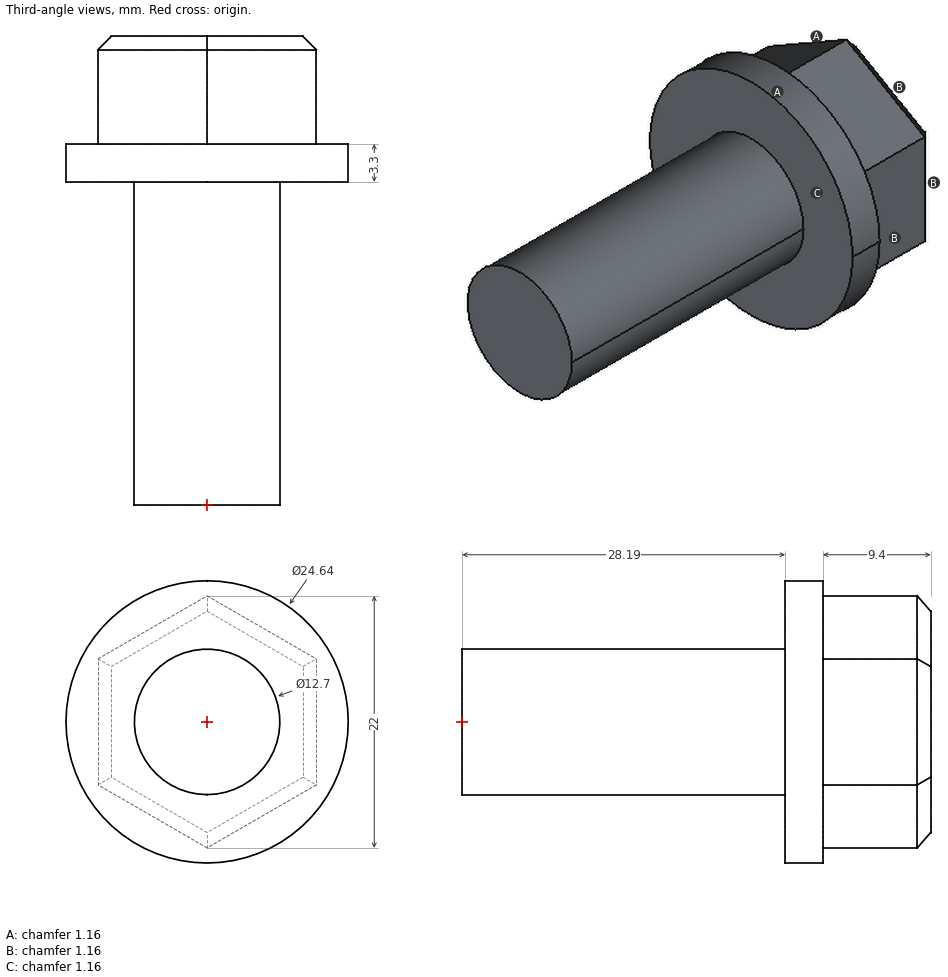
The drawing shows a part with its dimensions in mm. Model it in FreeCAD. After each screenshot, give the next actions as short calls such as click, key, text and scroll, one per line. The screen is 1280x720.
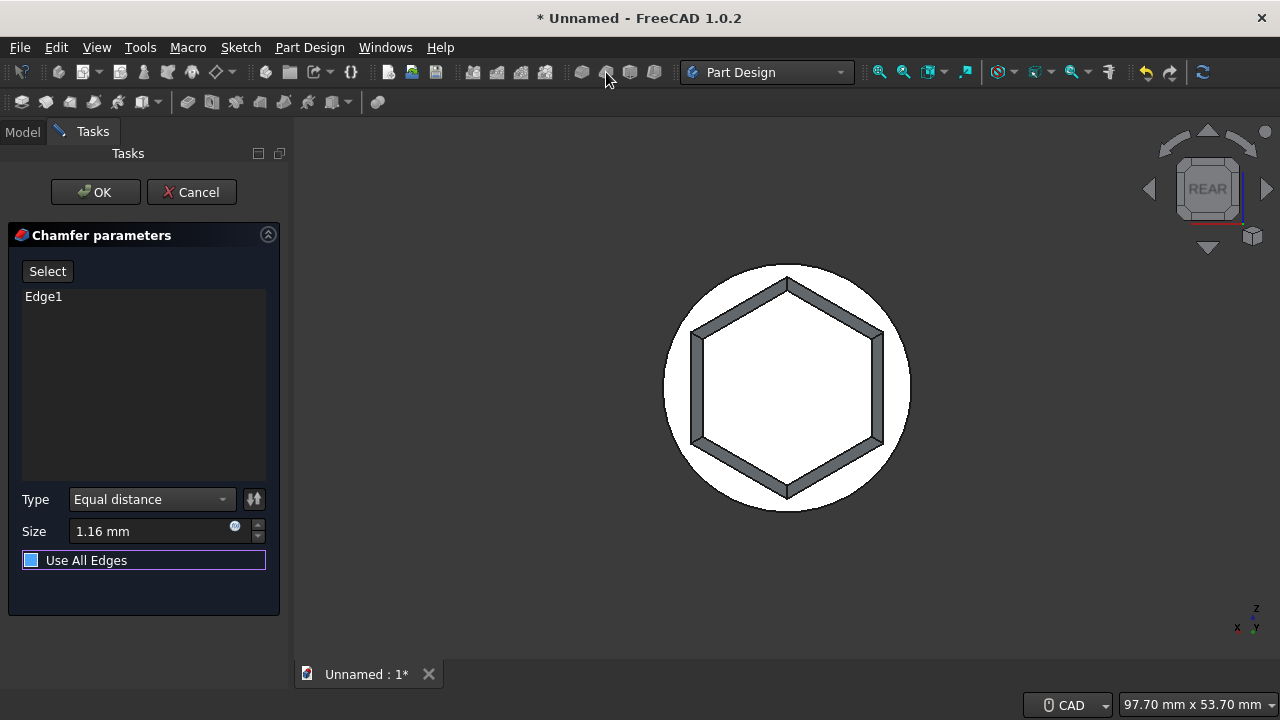
click(96, 192)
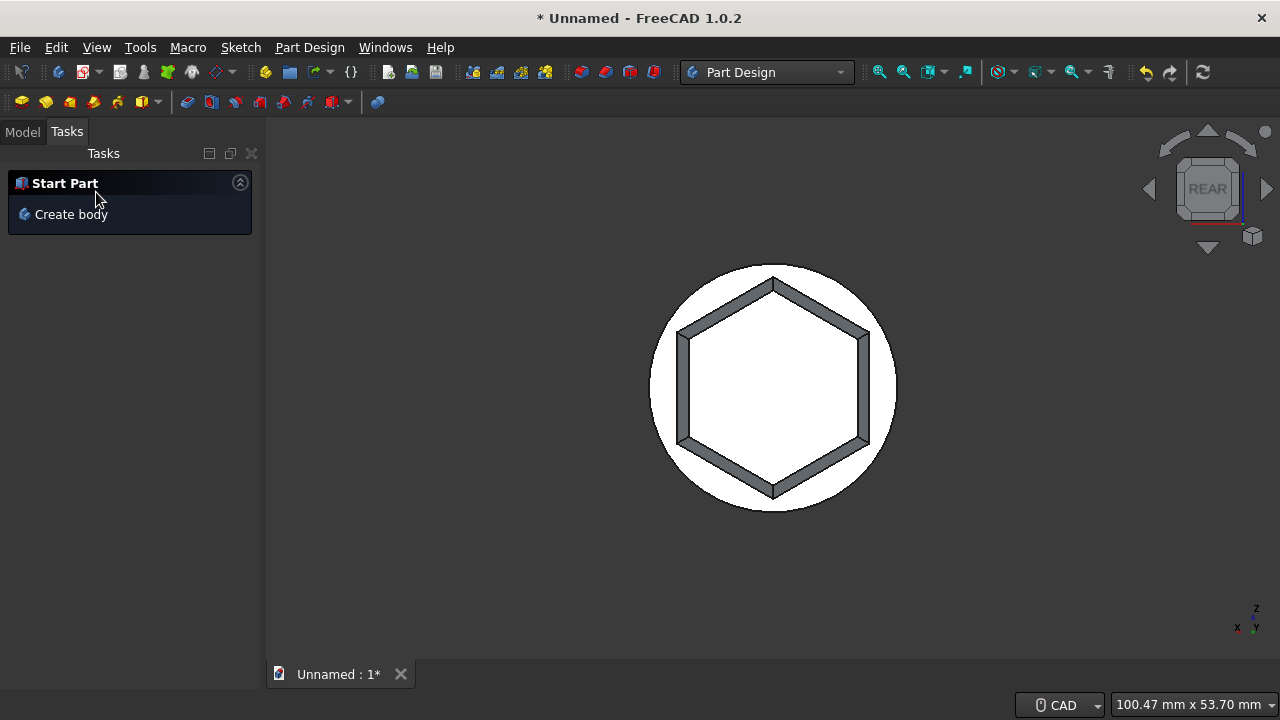
key(0)